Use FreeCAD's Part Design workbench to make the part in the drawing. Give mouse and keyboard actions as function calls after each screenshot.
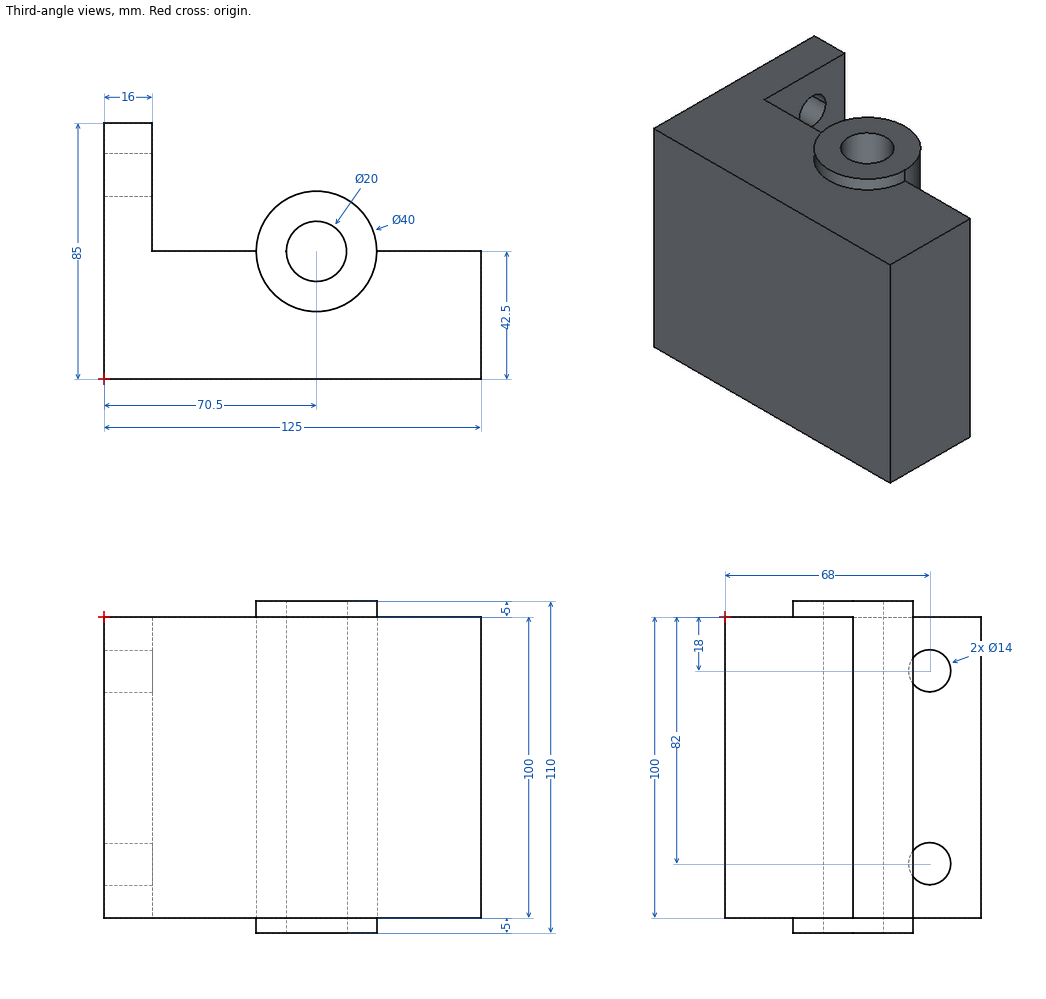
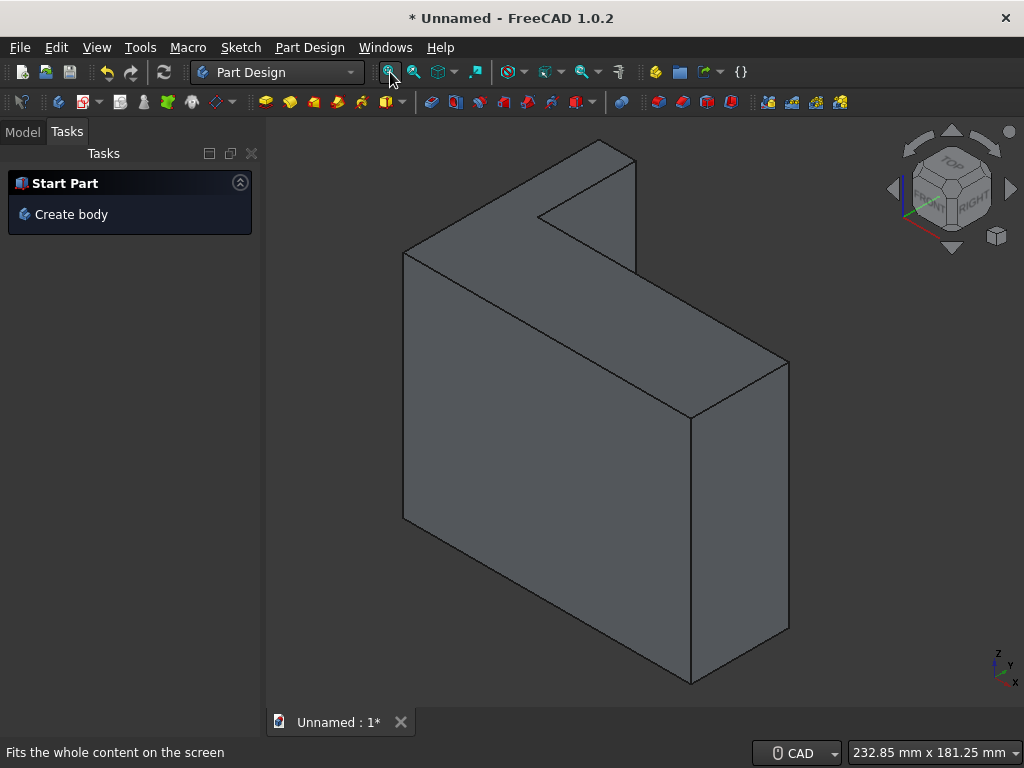
click(601, 237)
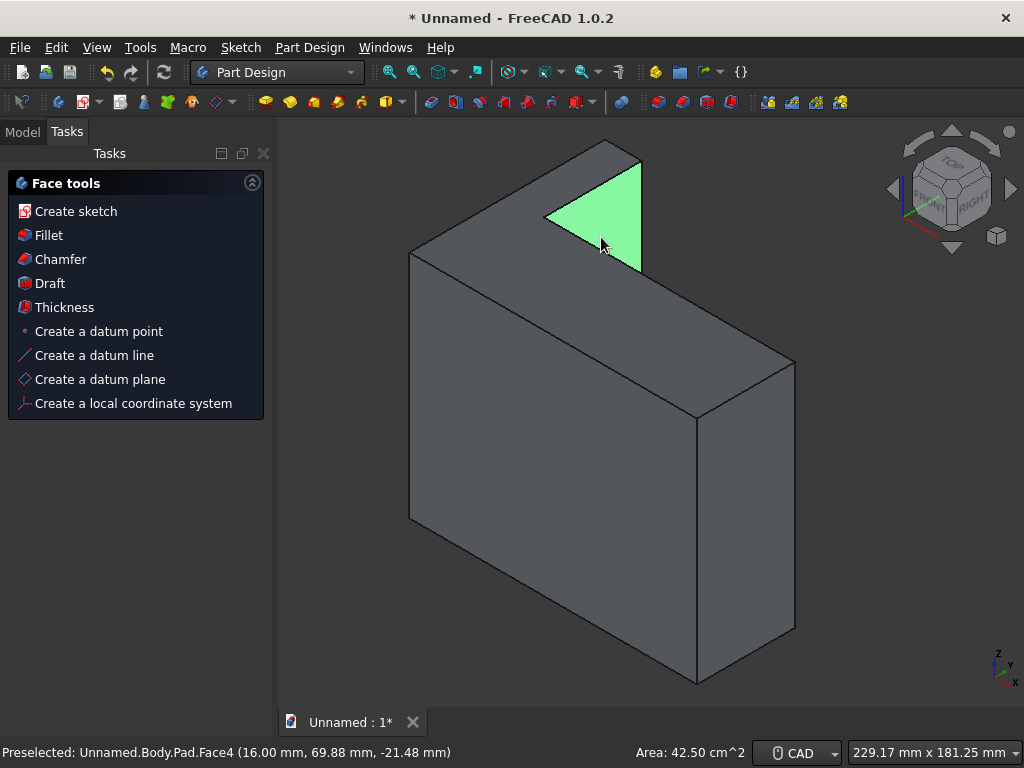
click(84, 102)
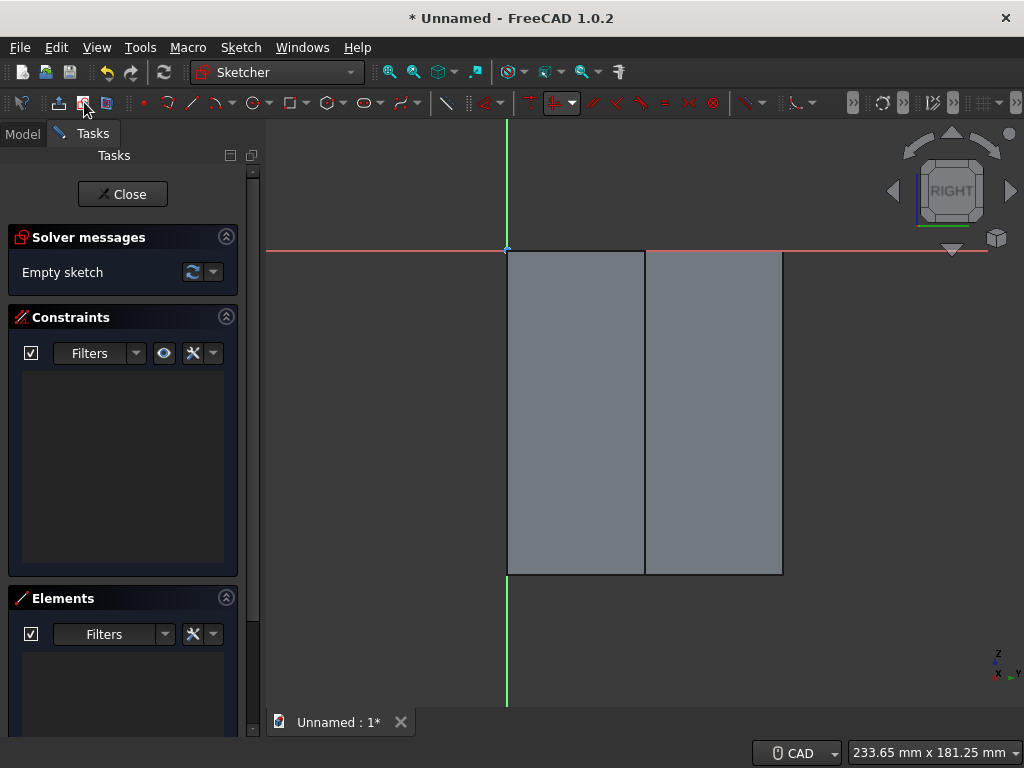
click(254, 104)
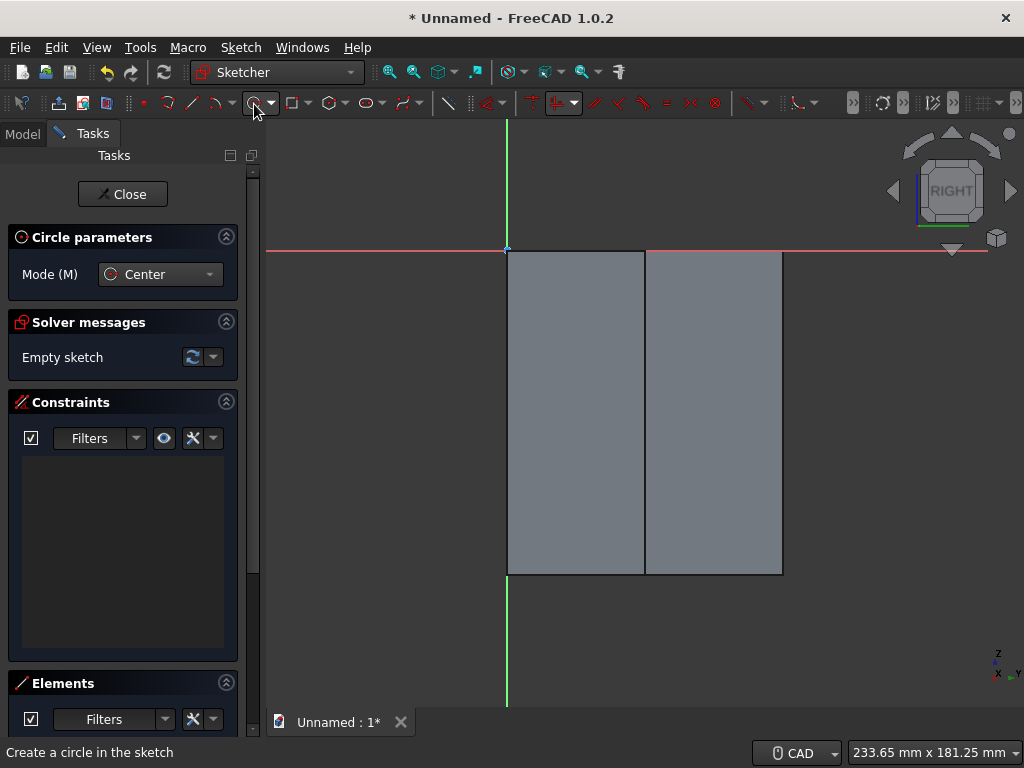
click(728, 309)
move(744, 293)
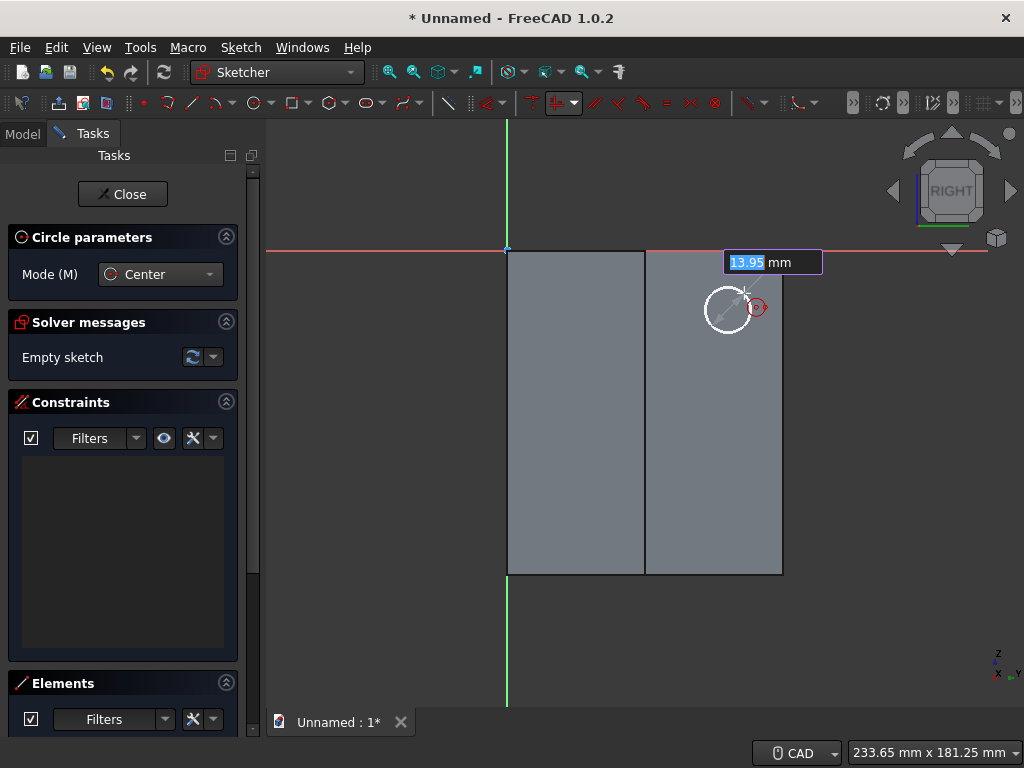
text(14)
key(Return)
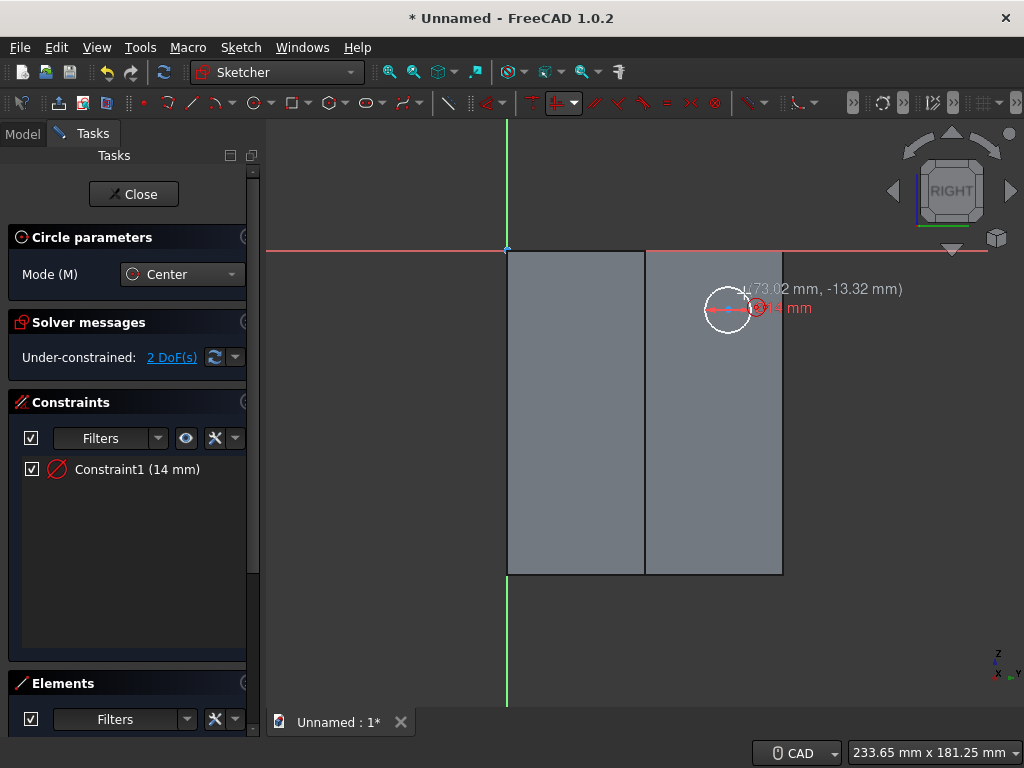
click(728, 517)
move(744, 501)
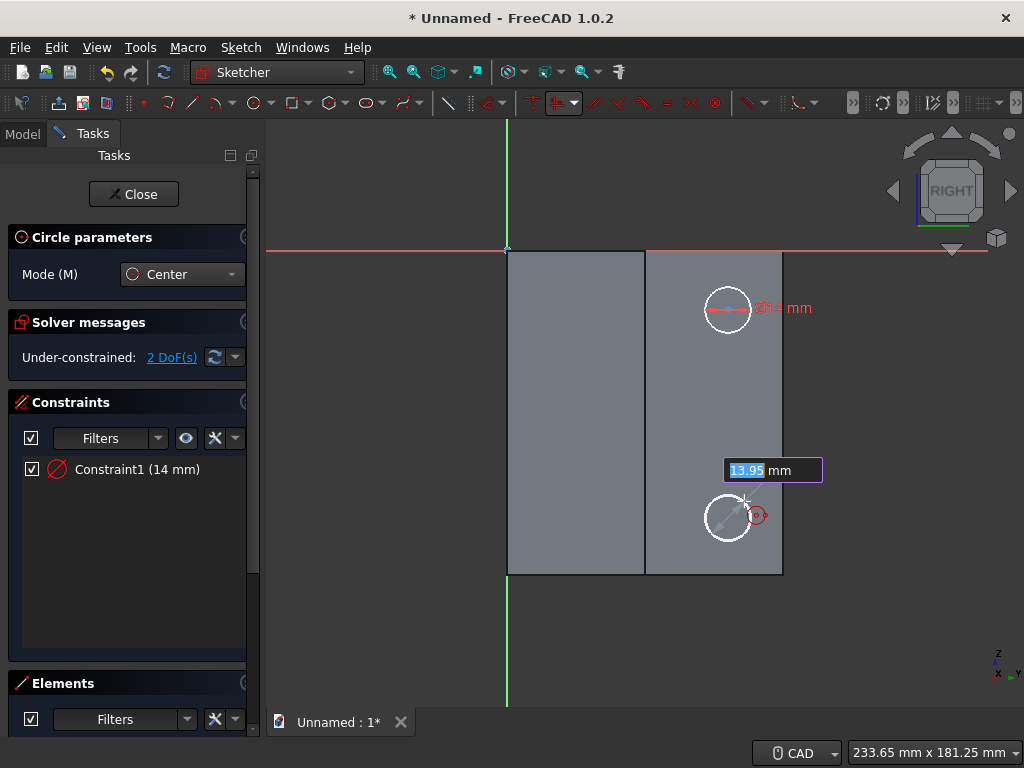
text(14)
key(Return)
key(Escape)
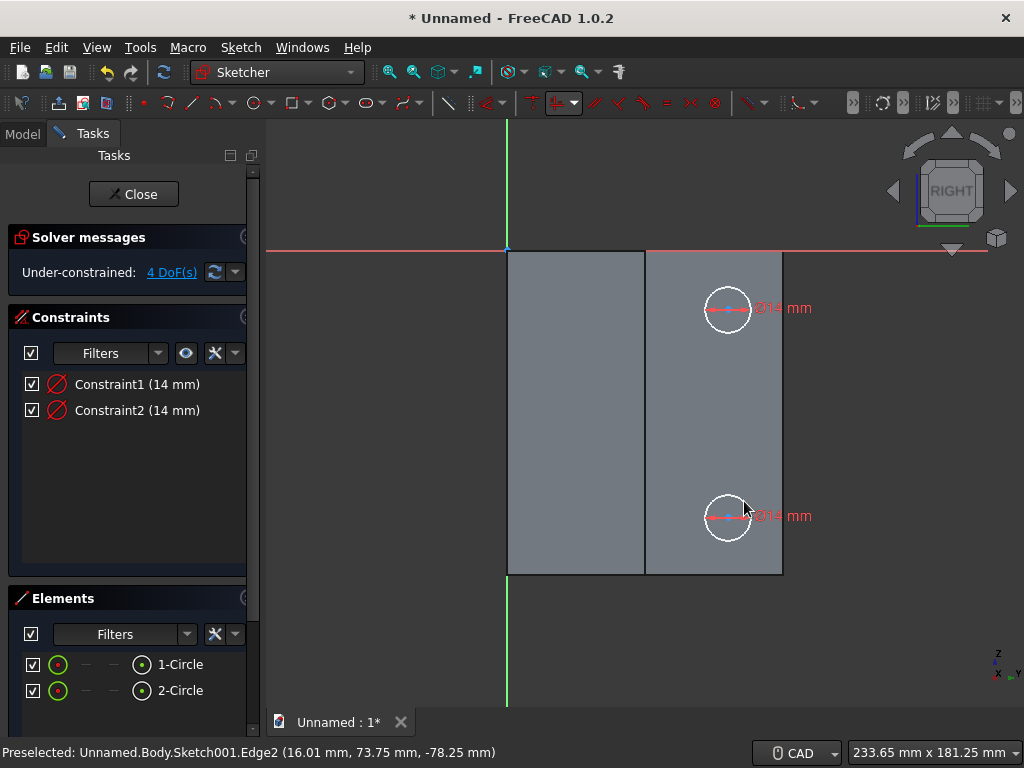
key(d)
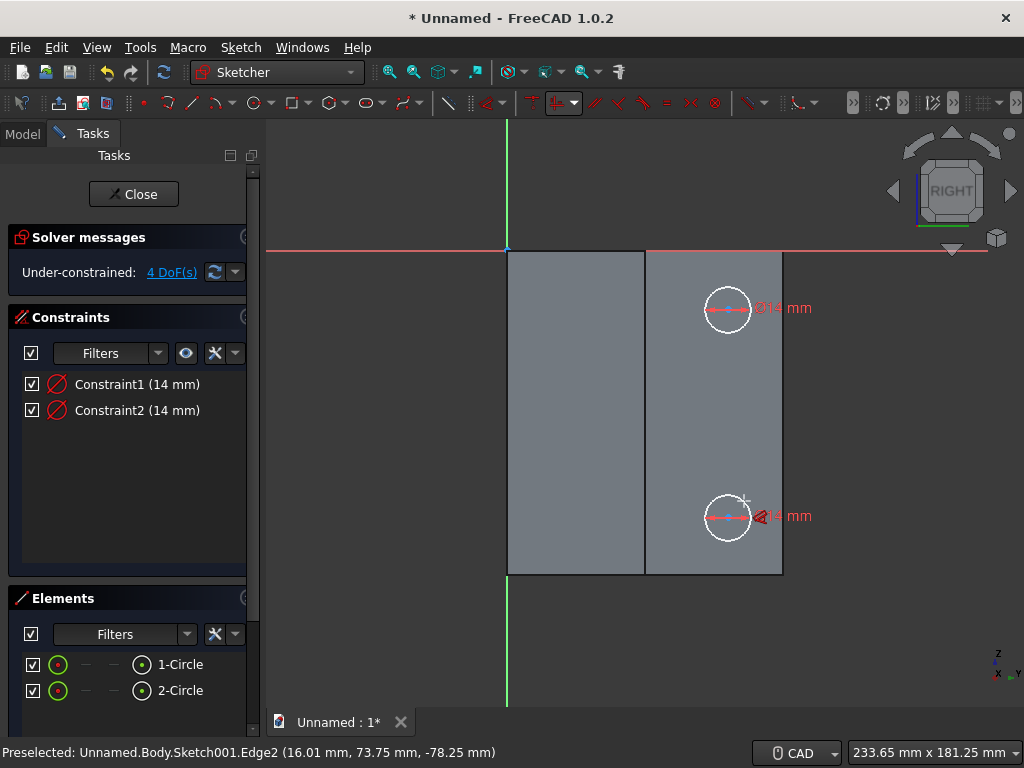
click(728, 310)
click(618, 217)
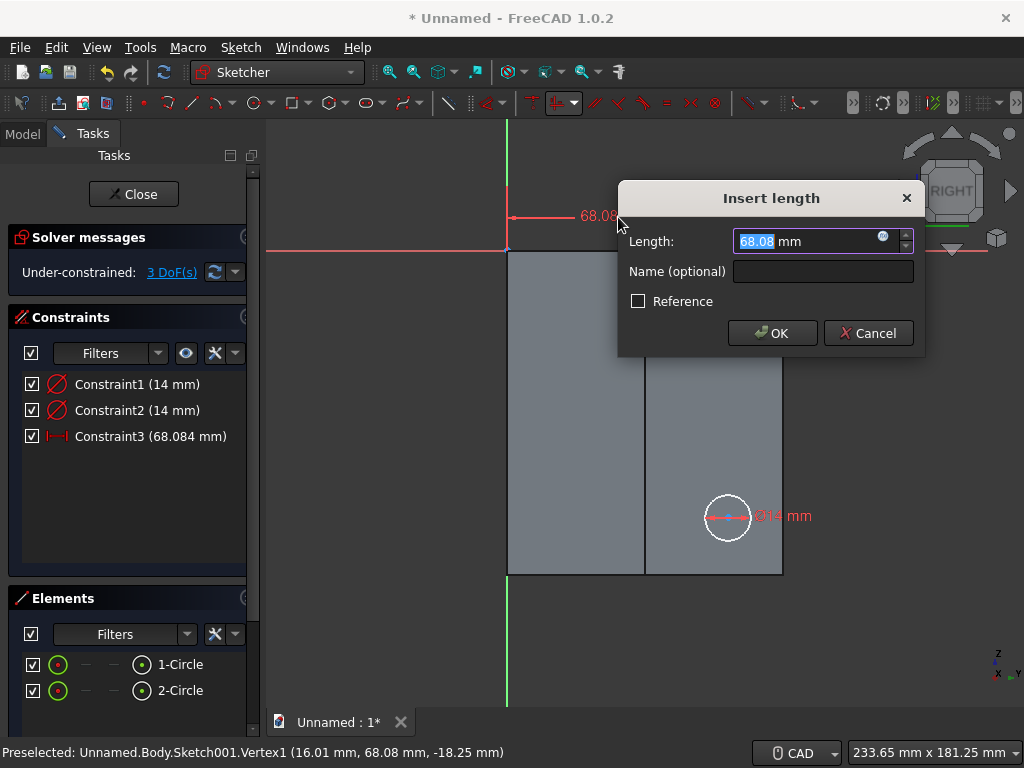
text(68)
key(Return)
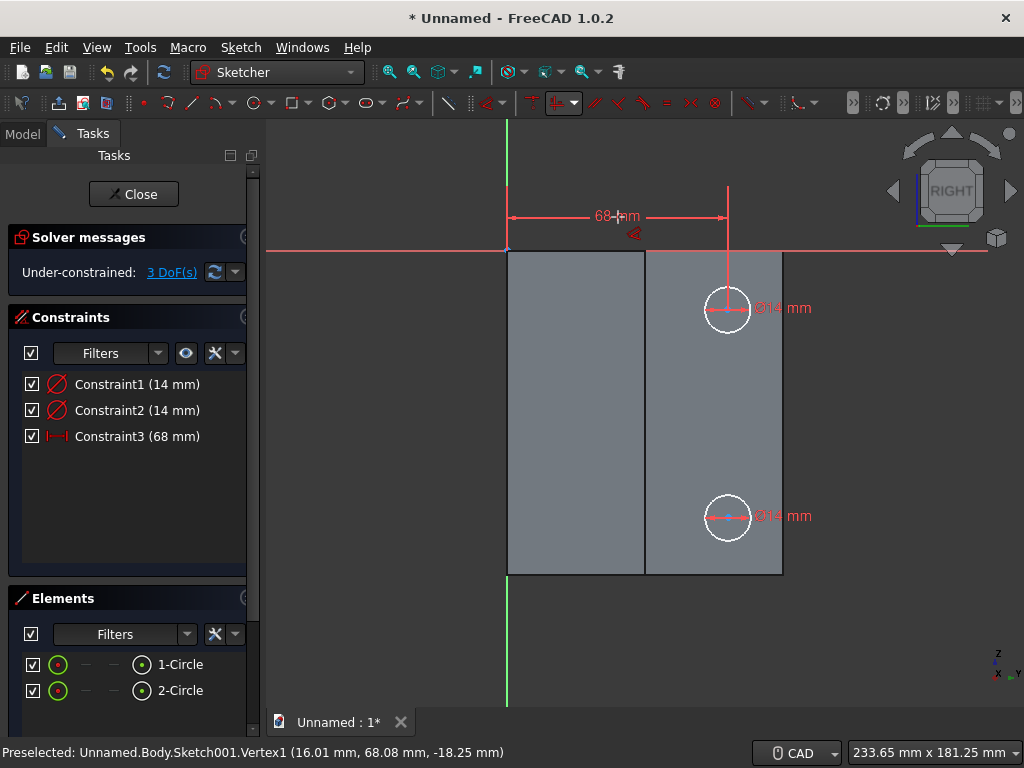
click(728, 310)
click(473, 280)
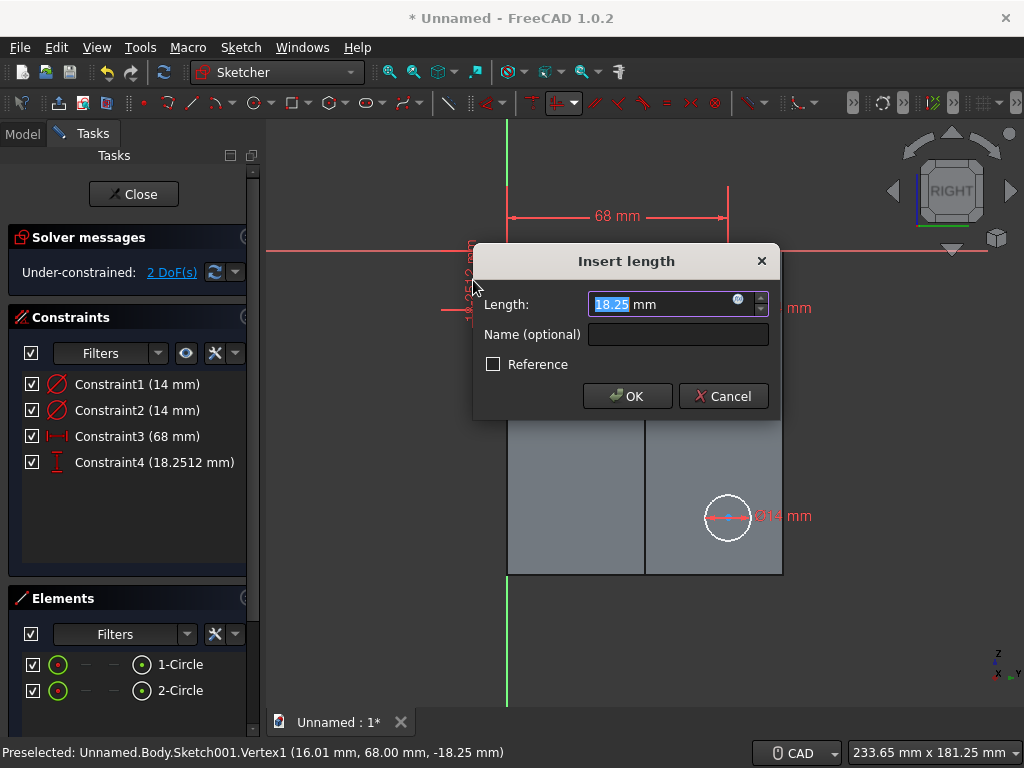
text(18)
key(Return)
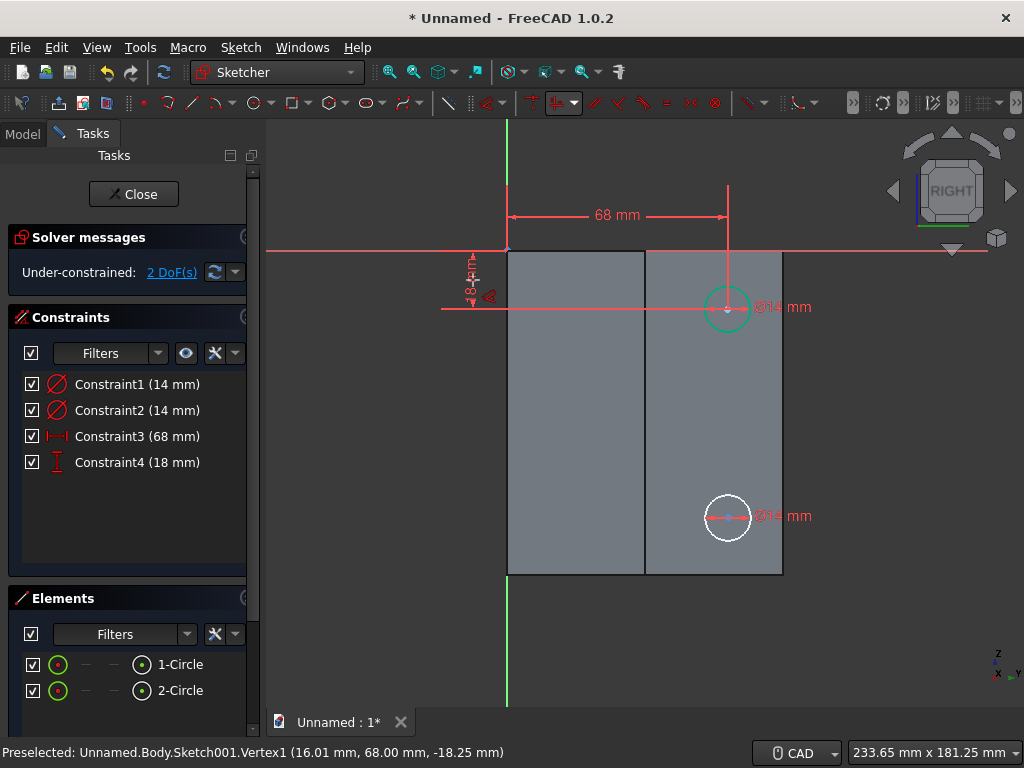
click(728, 518)
click(540, 217)